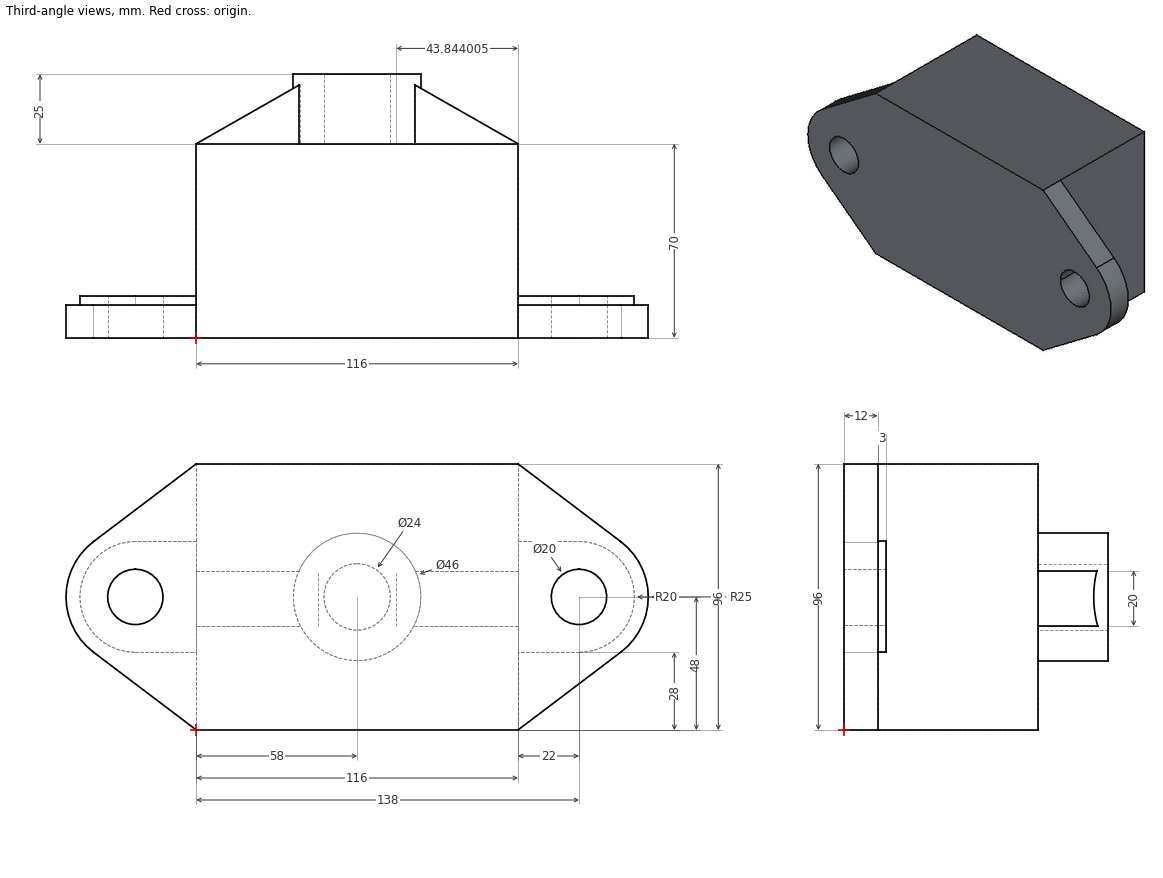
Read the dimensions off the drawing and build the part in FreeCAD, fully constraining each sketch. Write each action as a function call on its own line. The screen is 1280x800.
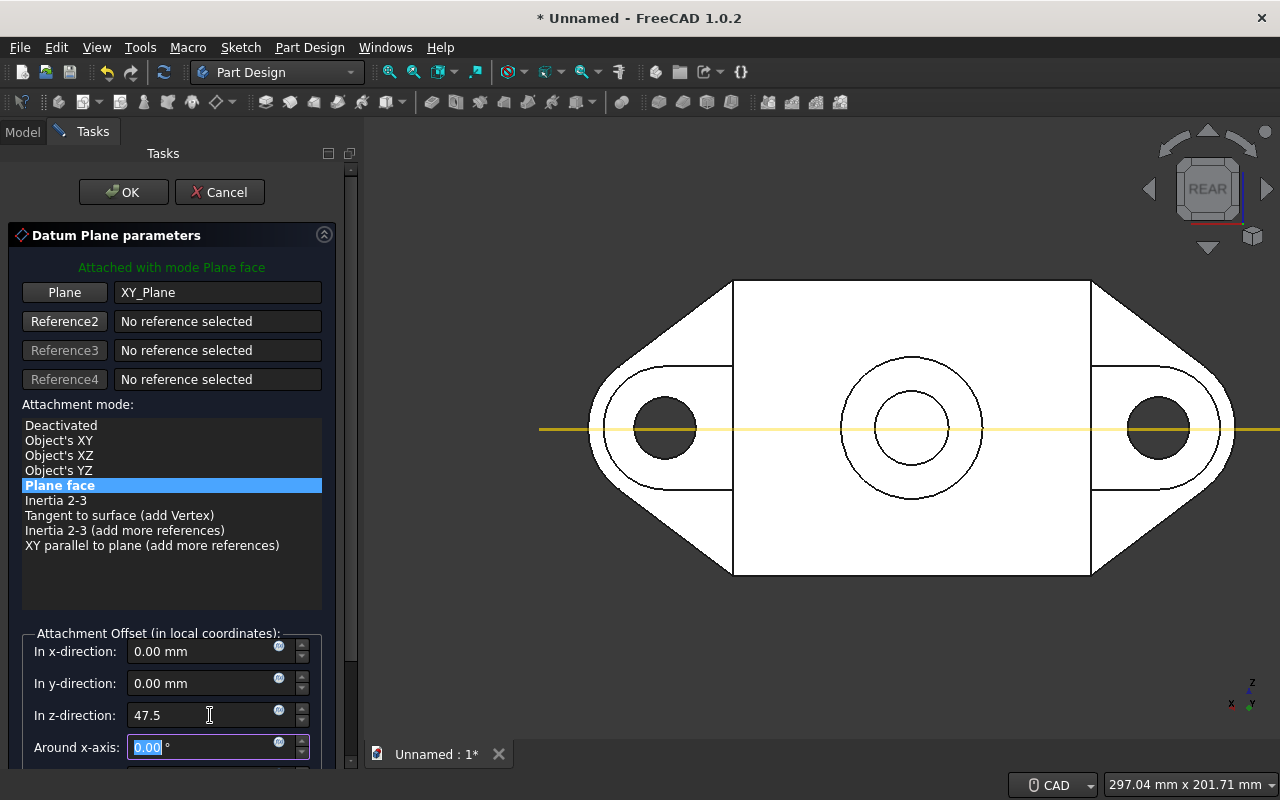
click(124, 192)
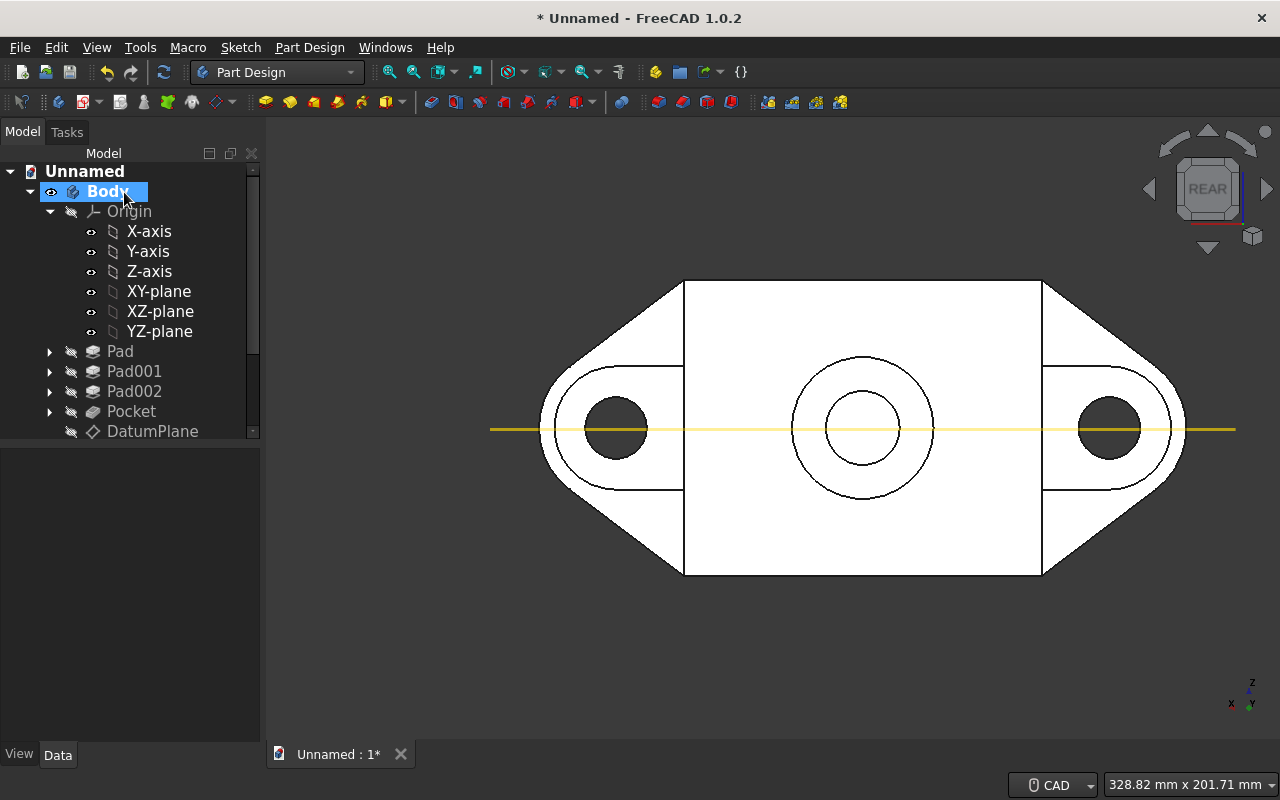
scroll(100, 307, down, 3)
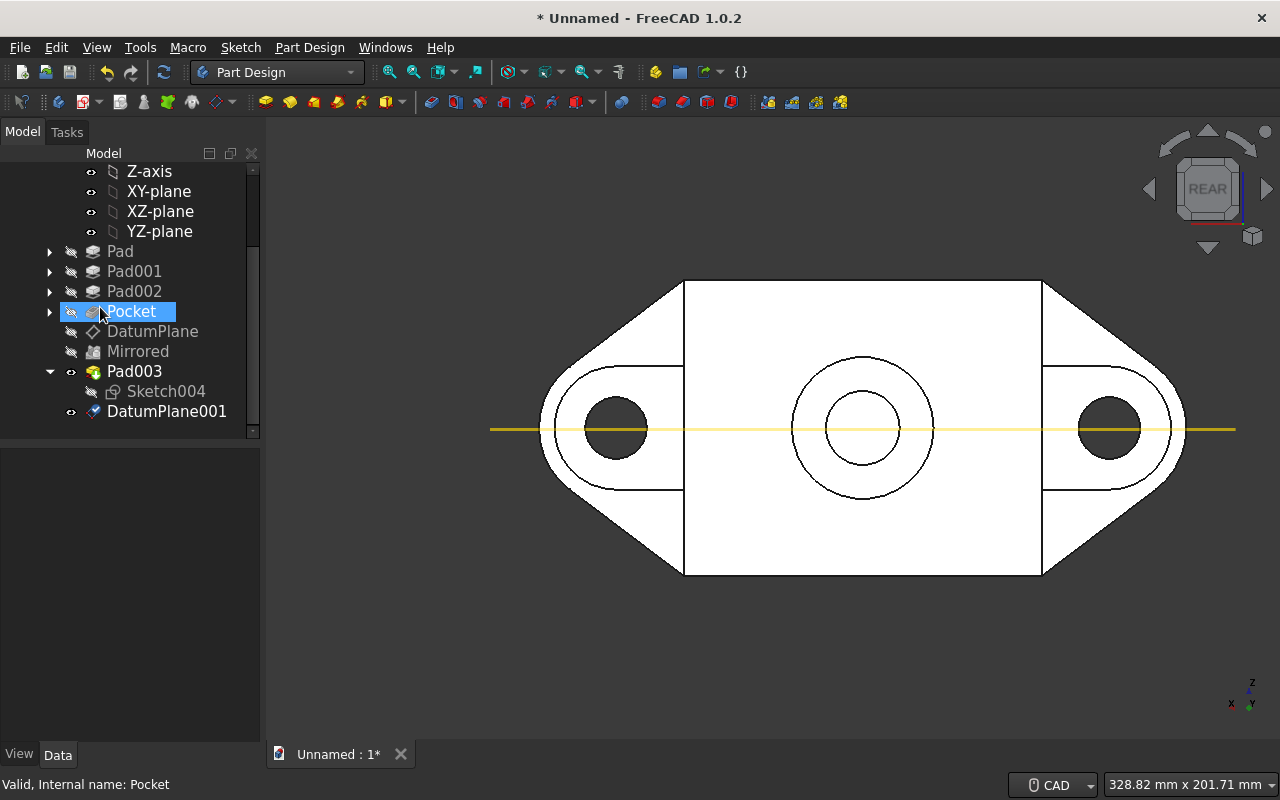
click(116, 412)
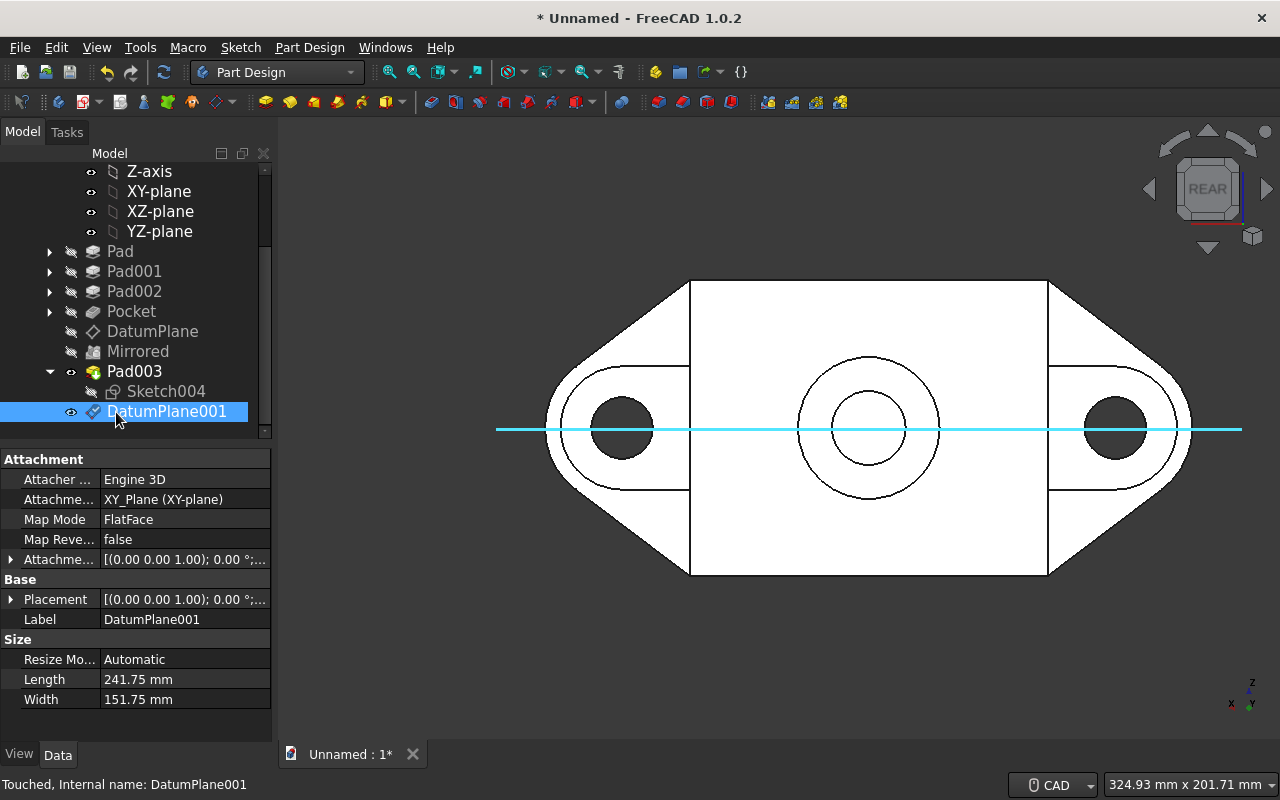
click(84, 102)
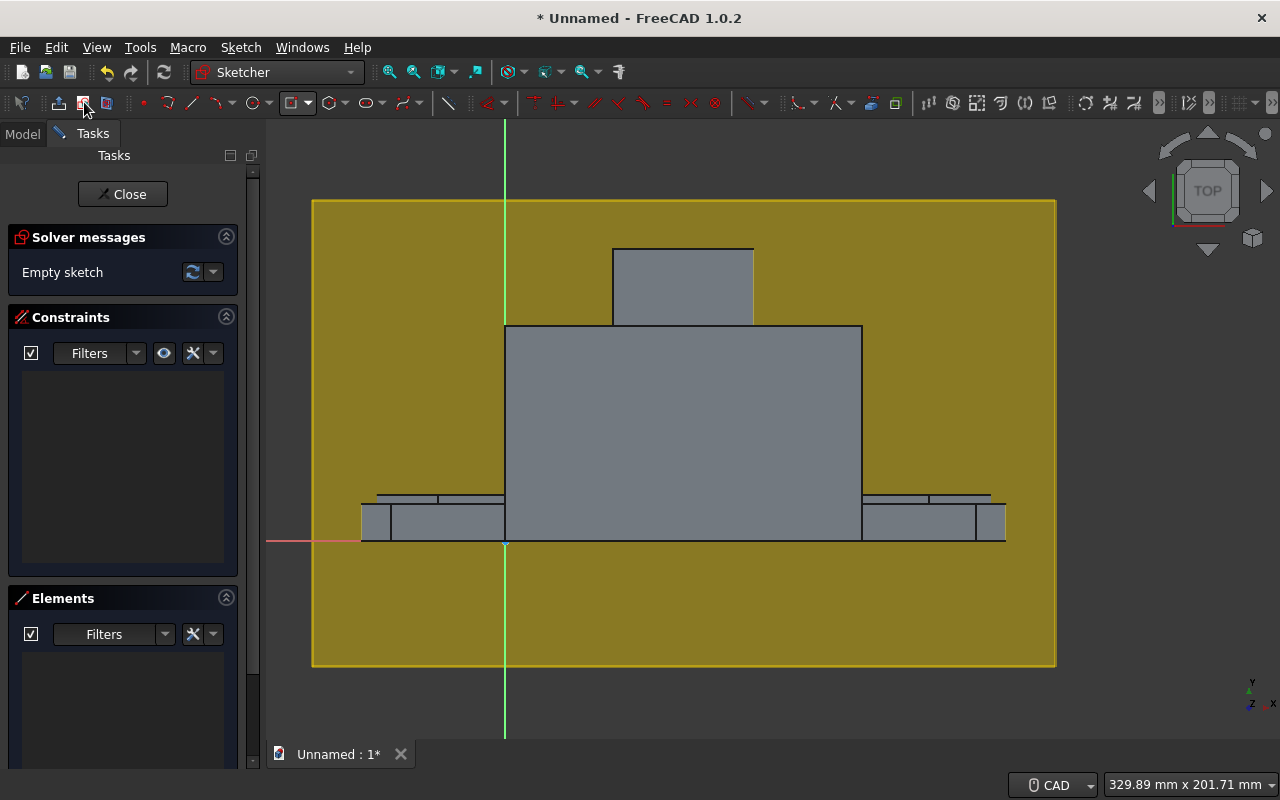
click(108, 104)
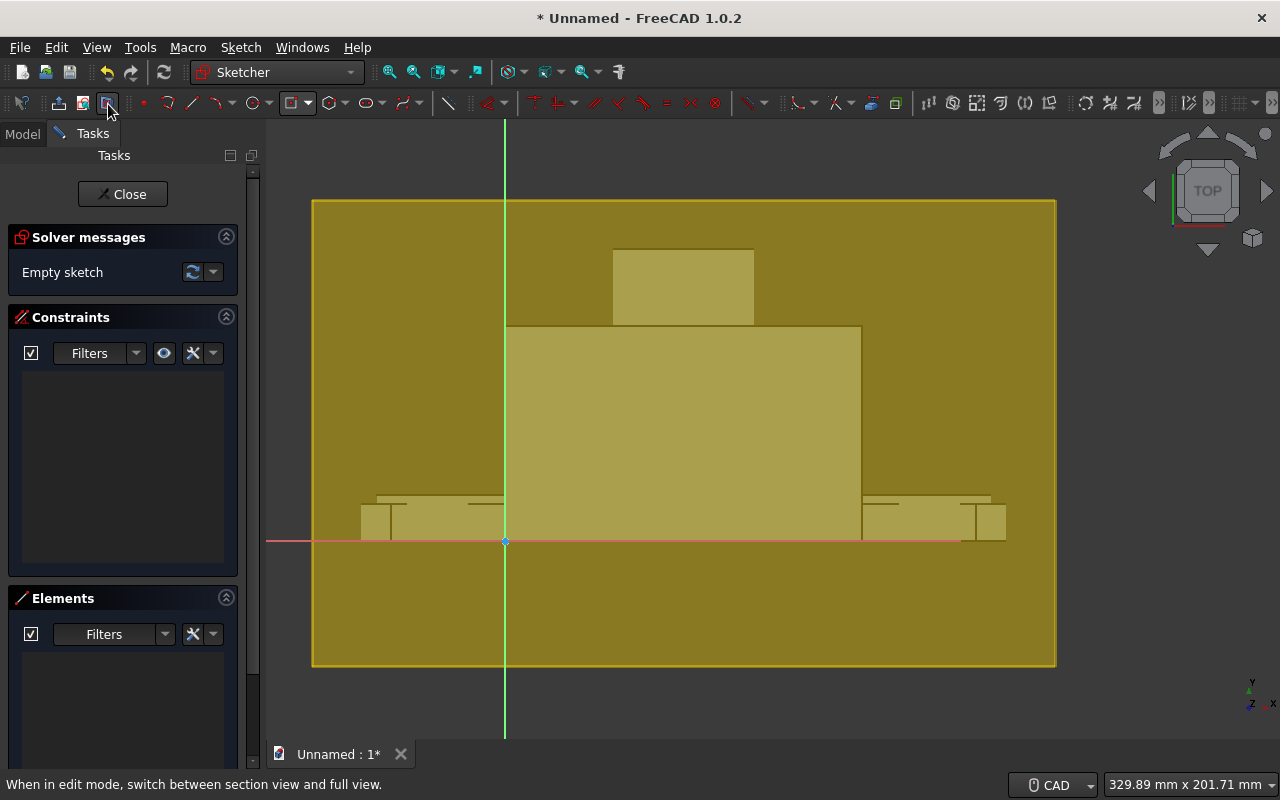
scroll(824, 241, up, 7)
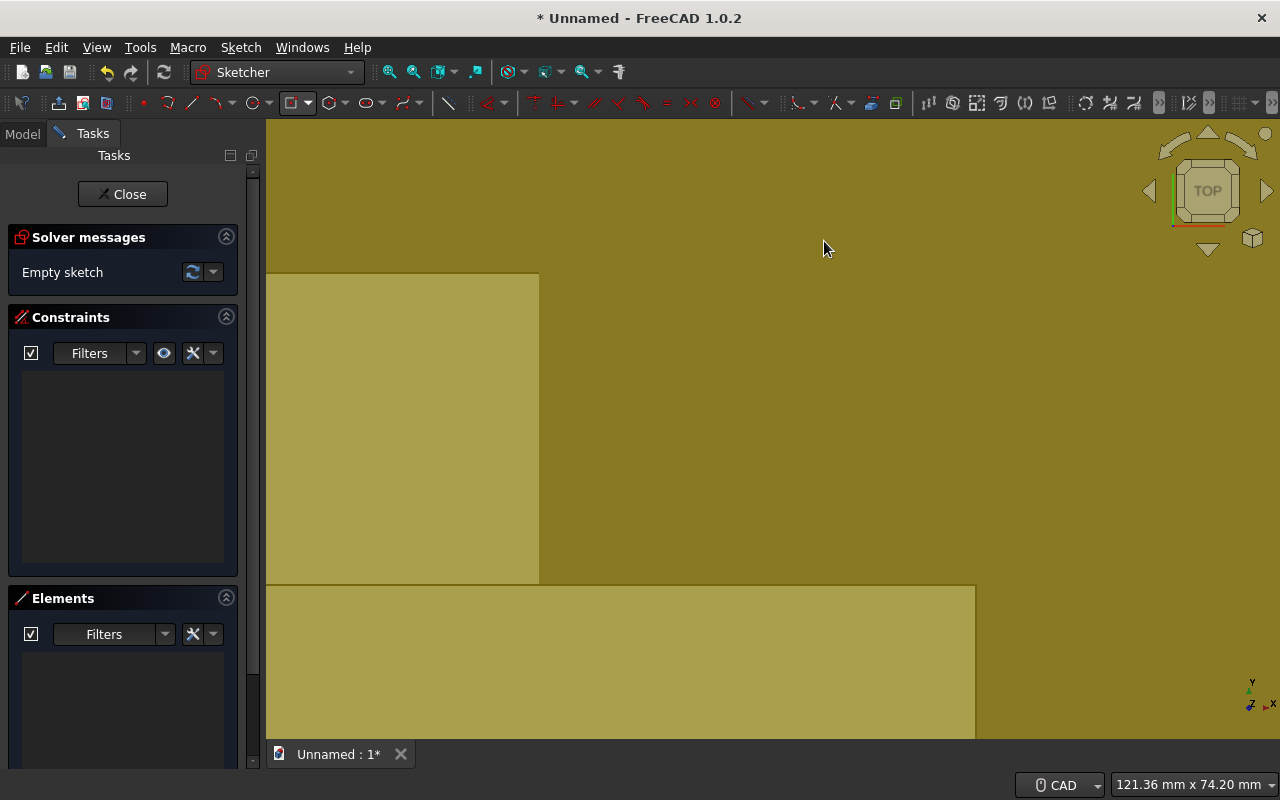
click(168, 104)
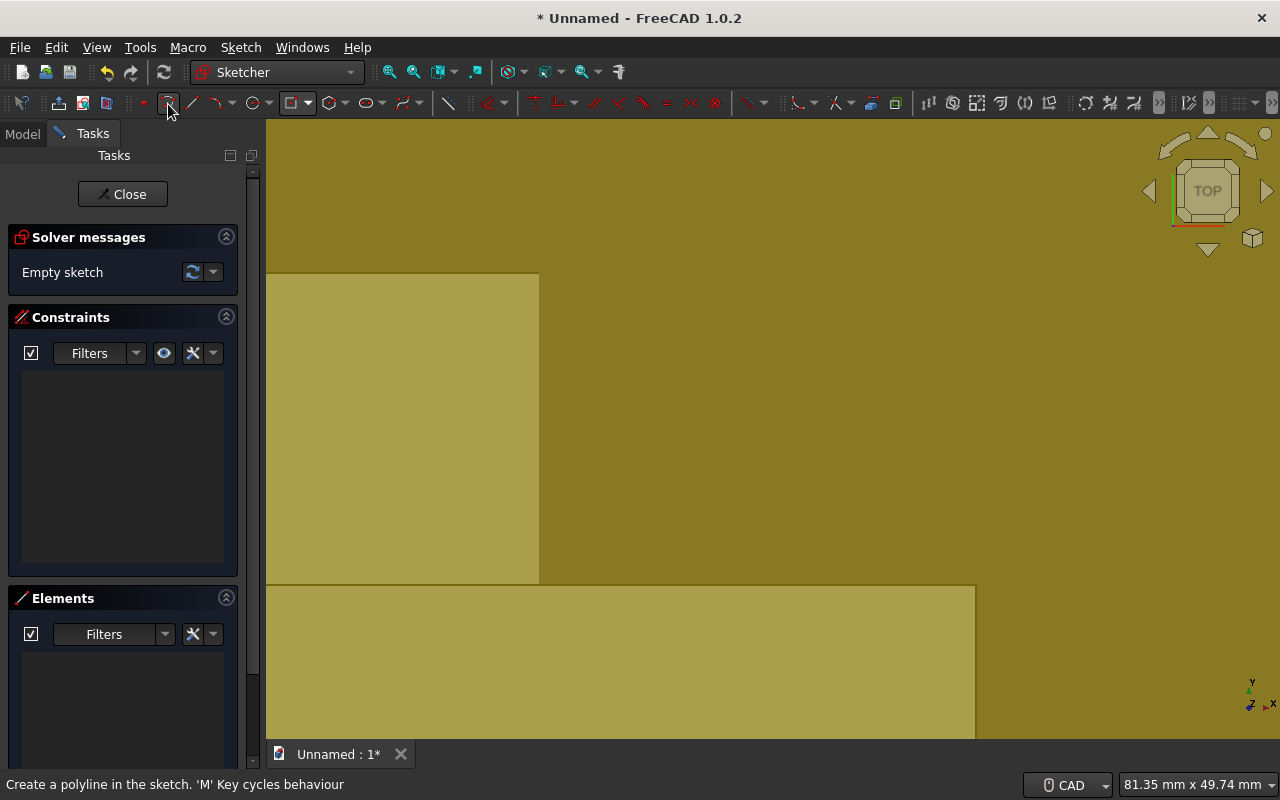
click(429, 585)
click(976, 585)
click(429, 273)
click(429, 586)
key(Escape)
key(Escape)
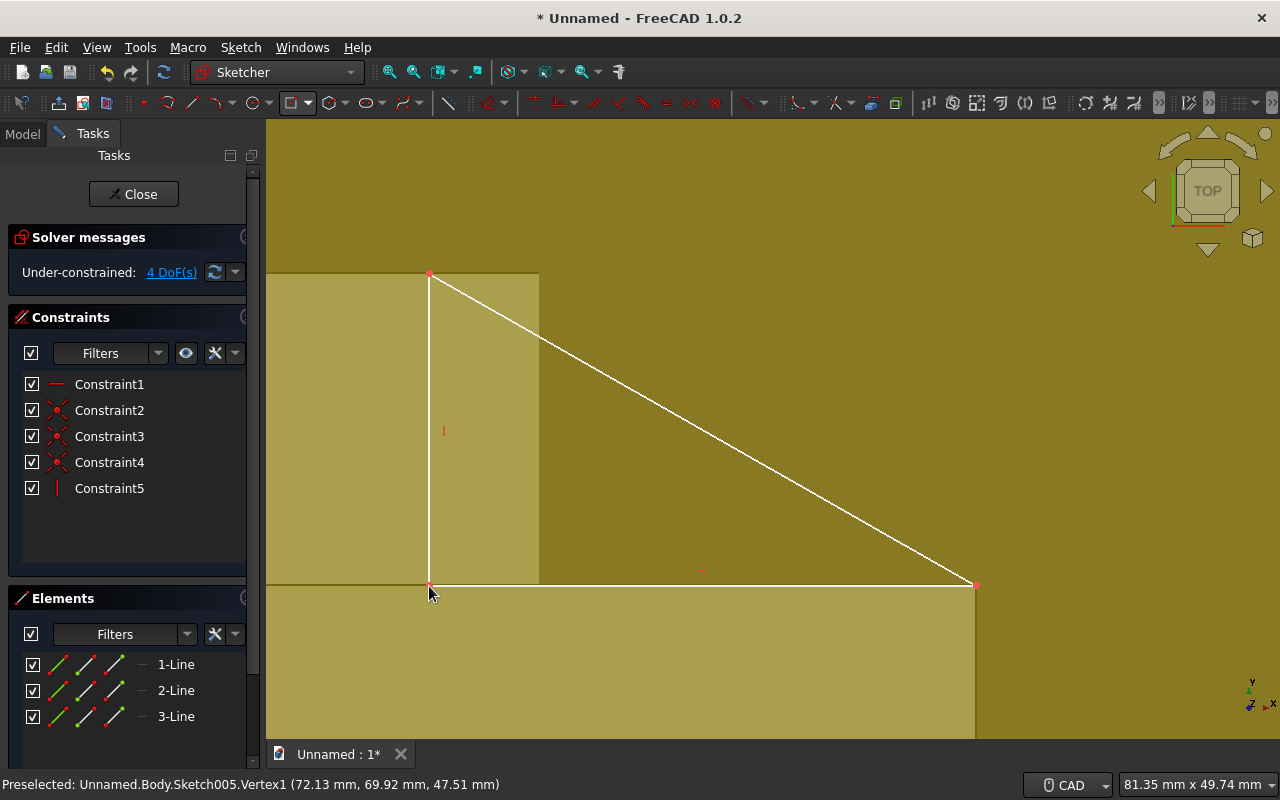
click(488, 104)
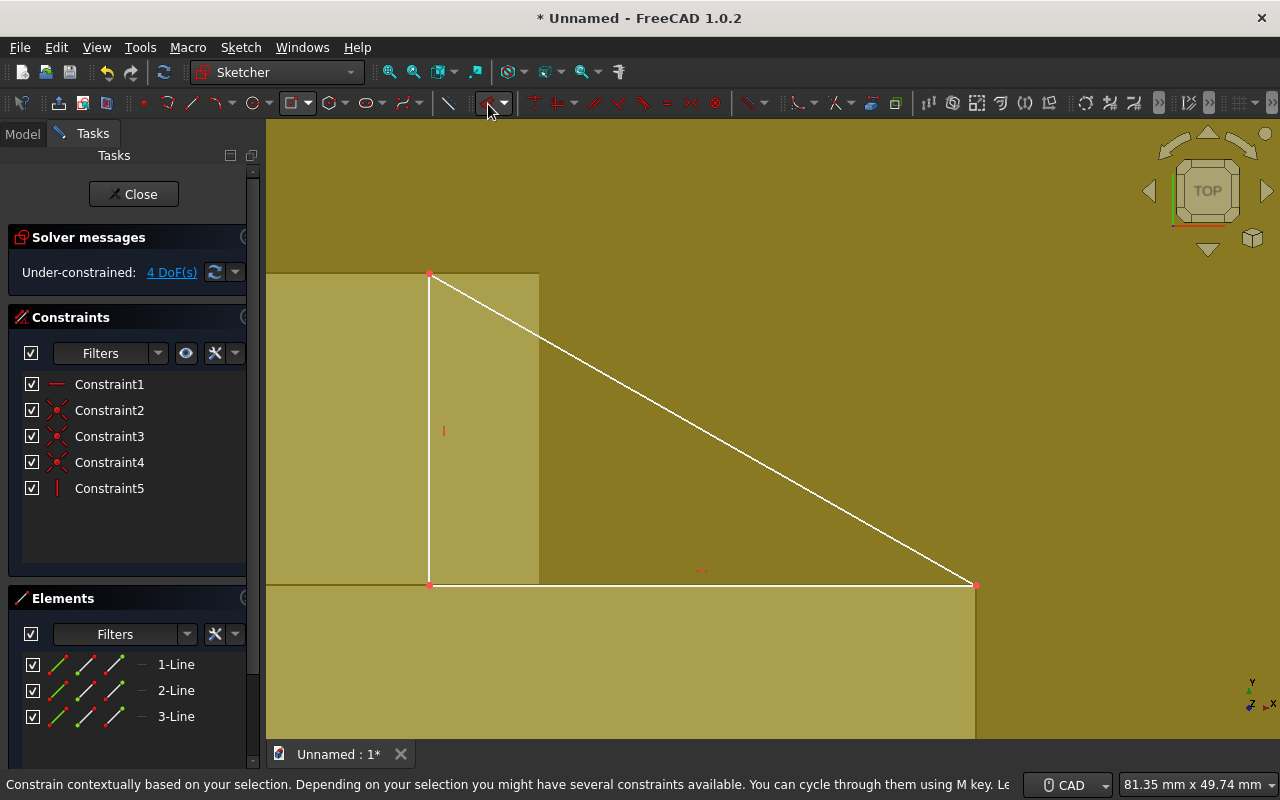
click(429, 368)
click(395, 430)